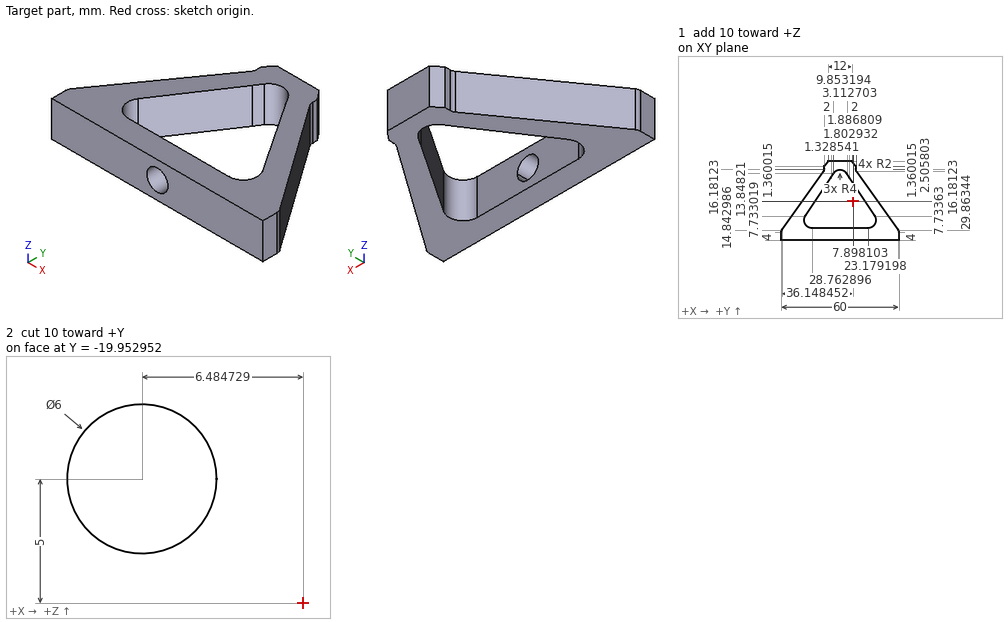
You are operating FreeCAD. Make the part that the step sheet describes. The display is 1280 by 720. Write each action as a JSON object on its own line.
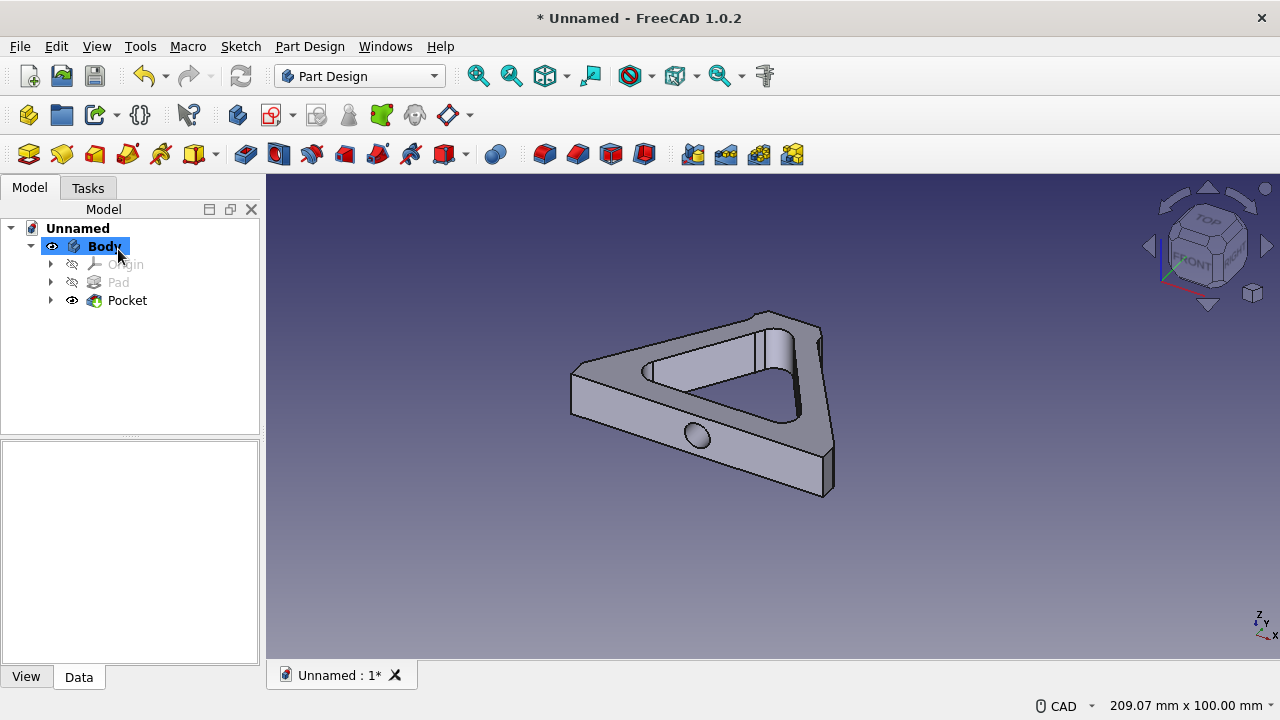
{"action": "key", "text": "0"}